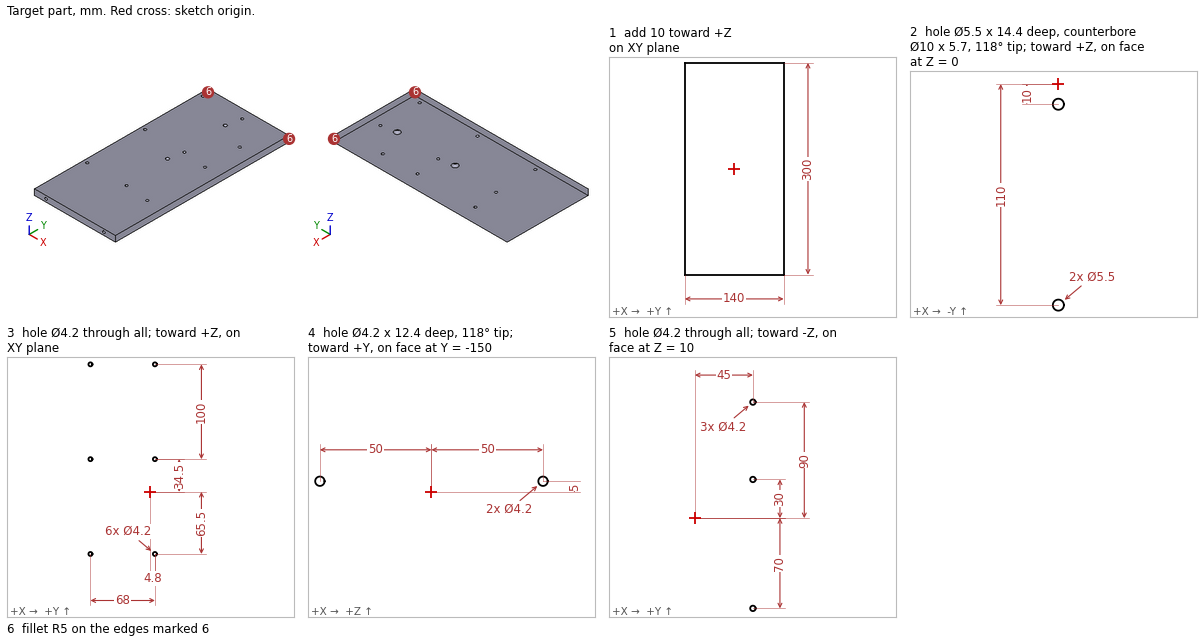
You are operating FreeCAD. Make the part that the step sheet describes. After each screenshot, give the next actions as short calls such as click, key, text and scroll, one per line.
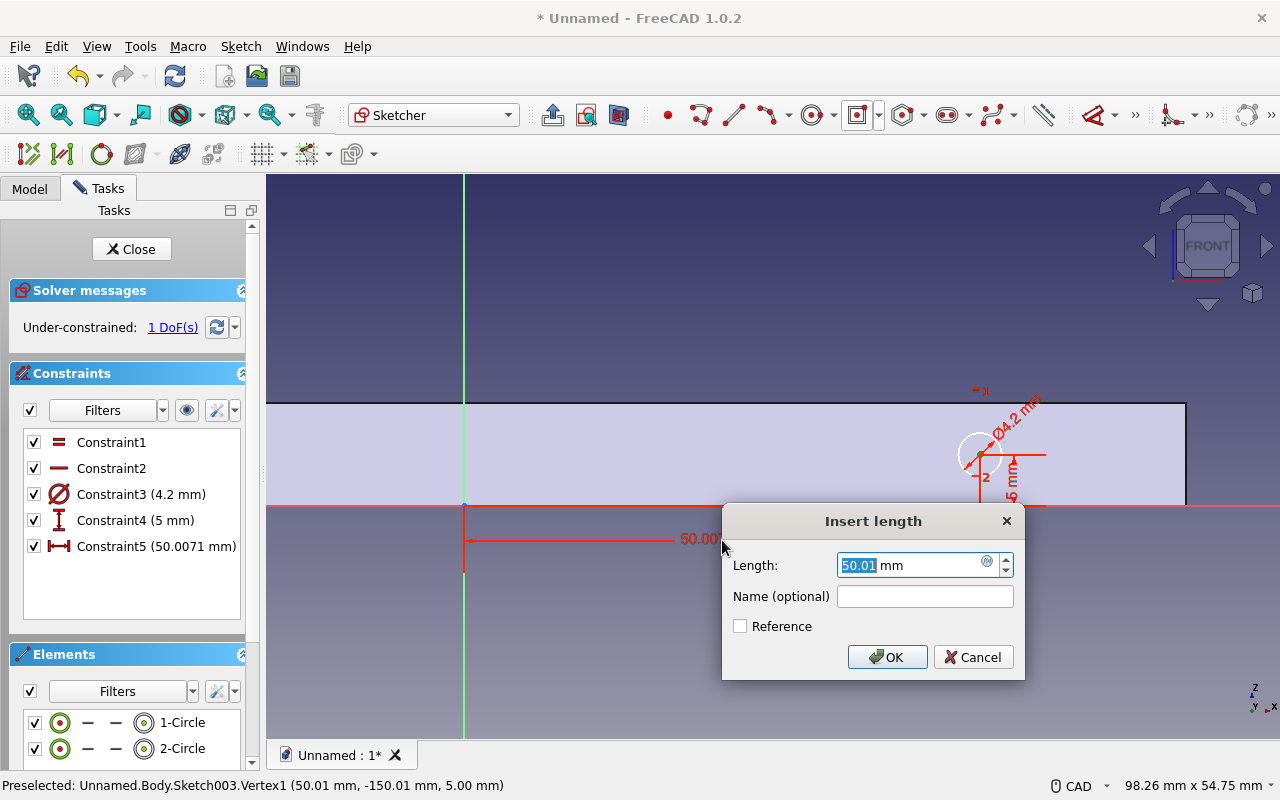
text(50)
key(Return)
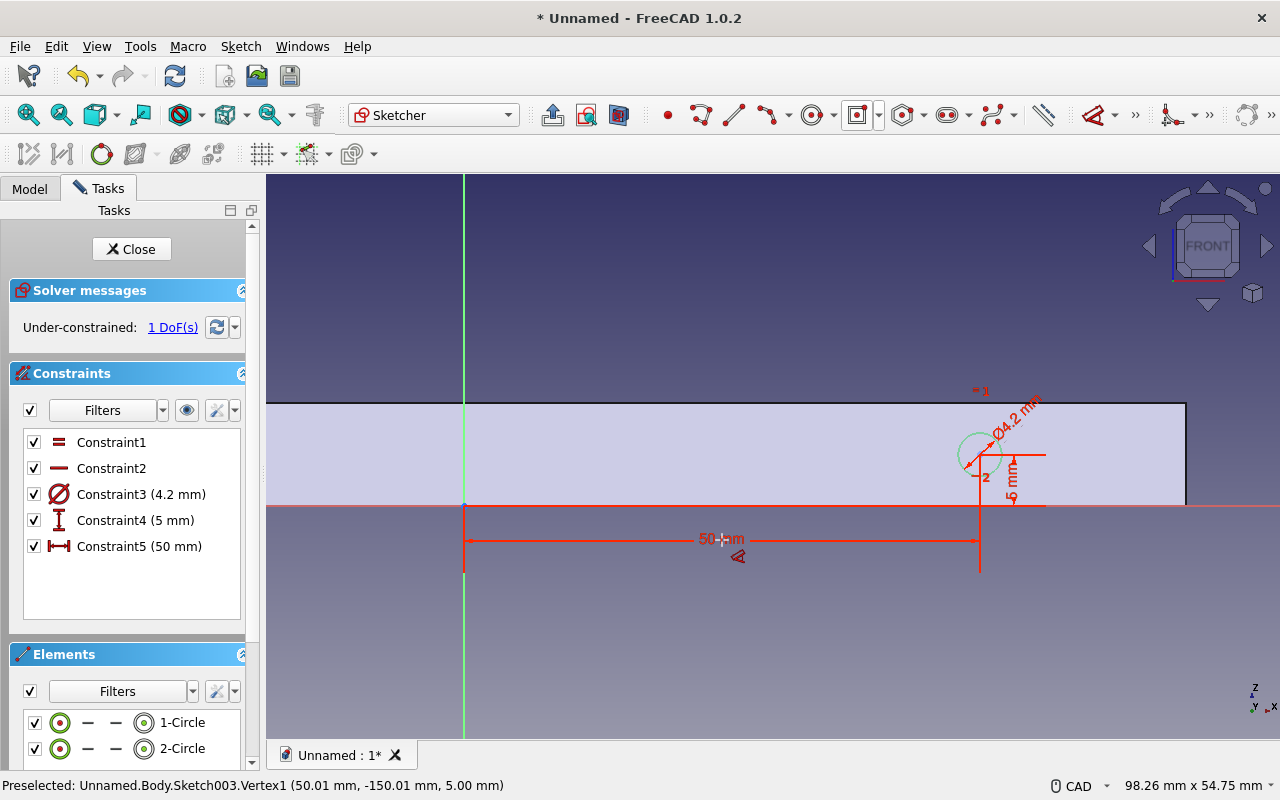
scroll(997, 440, down, 3)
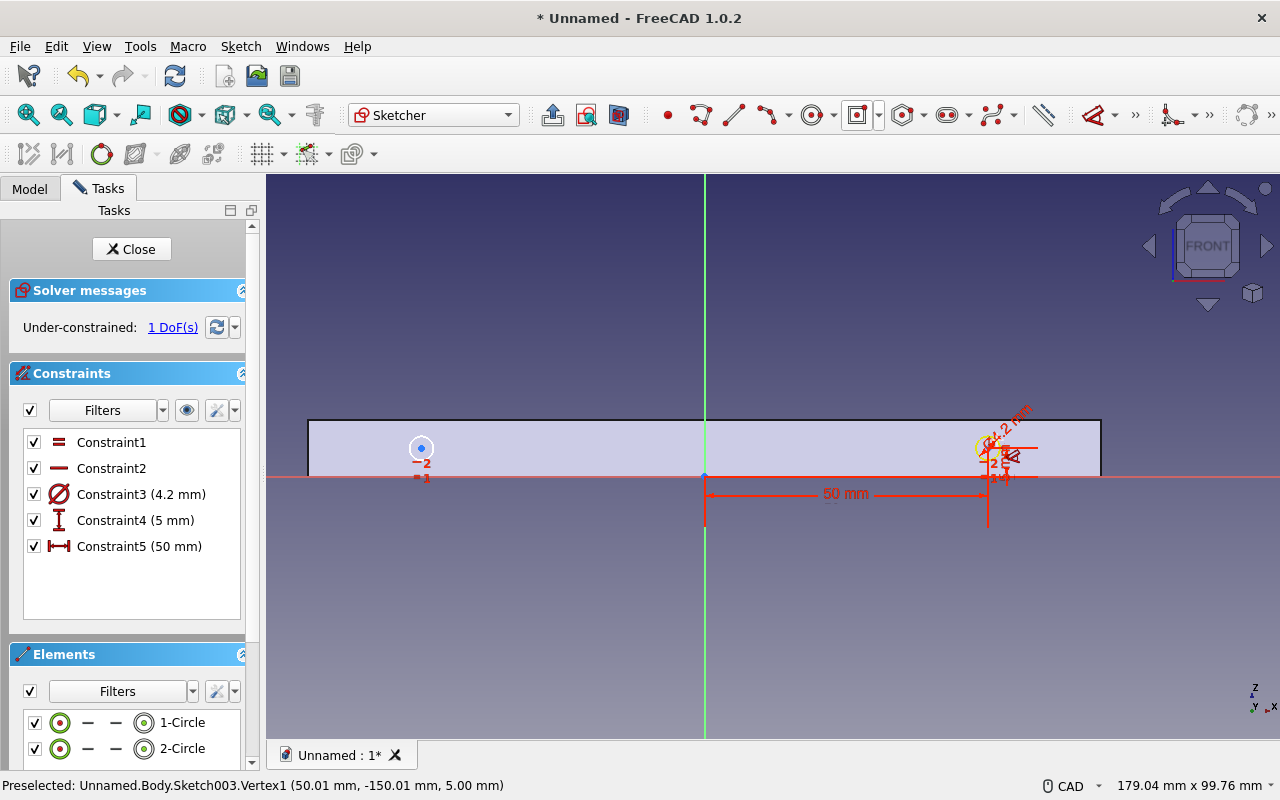
click(422, 448)
click(563, 511)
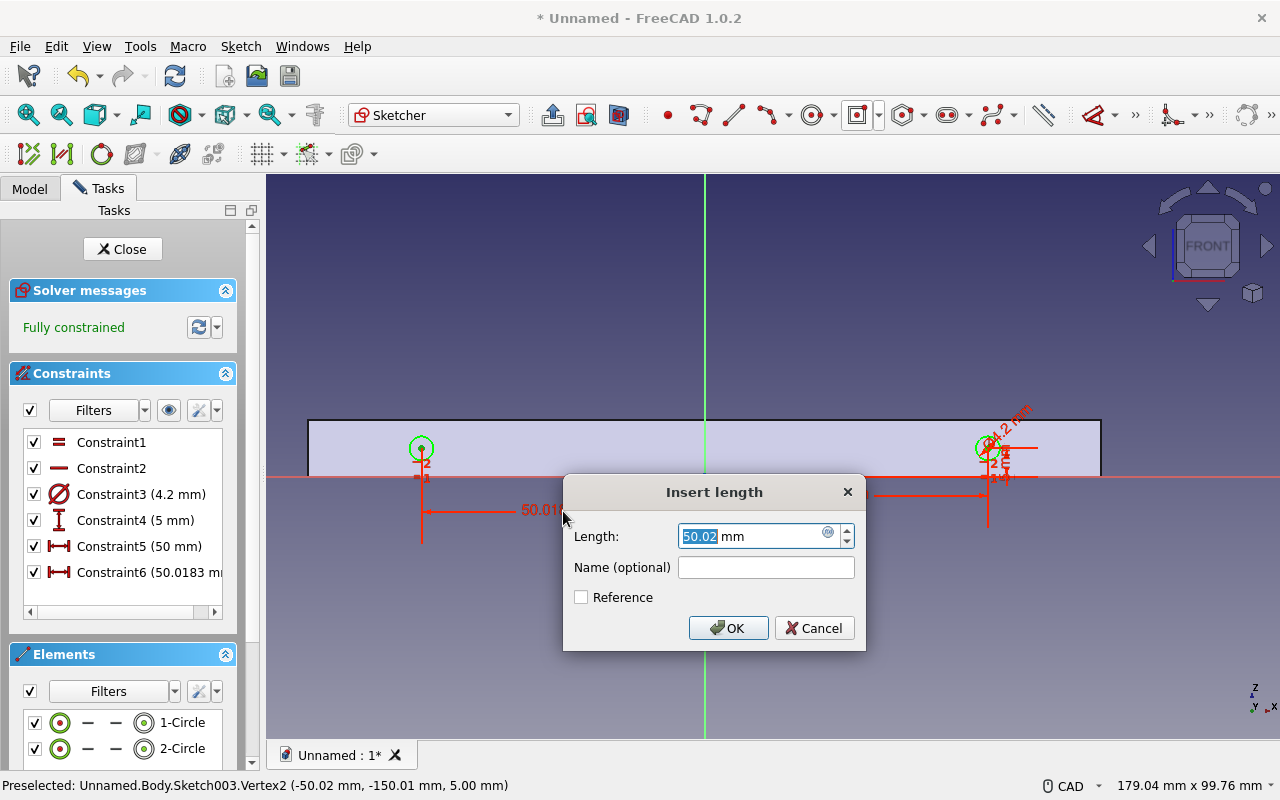
text(50)
key(Return)
key(Escape)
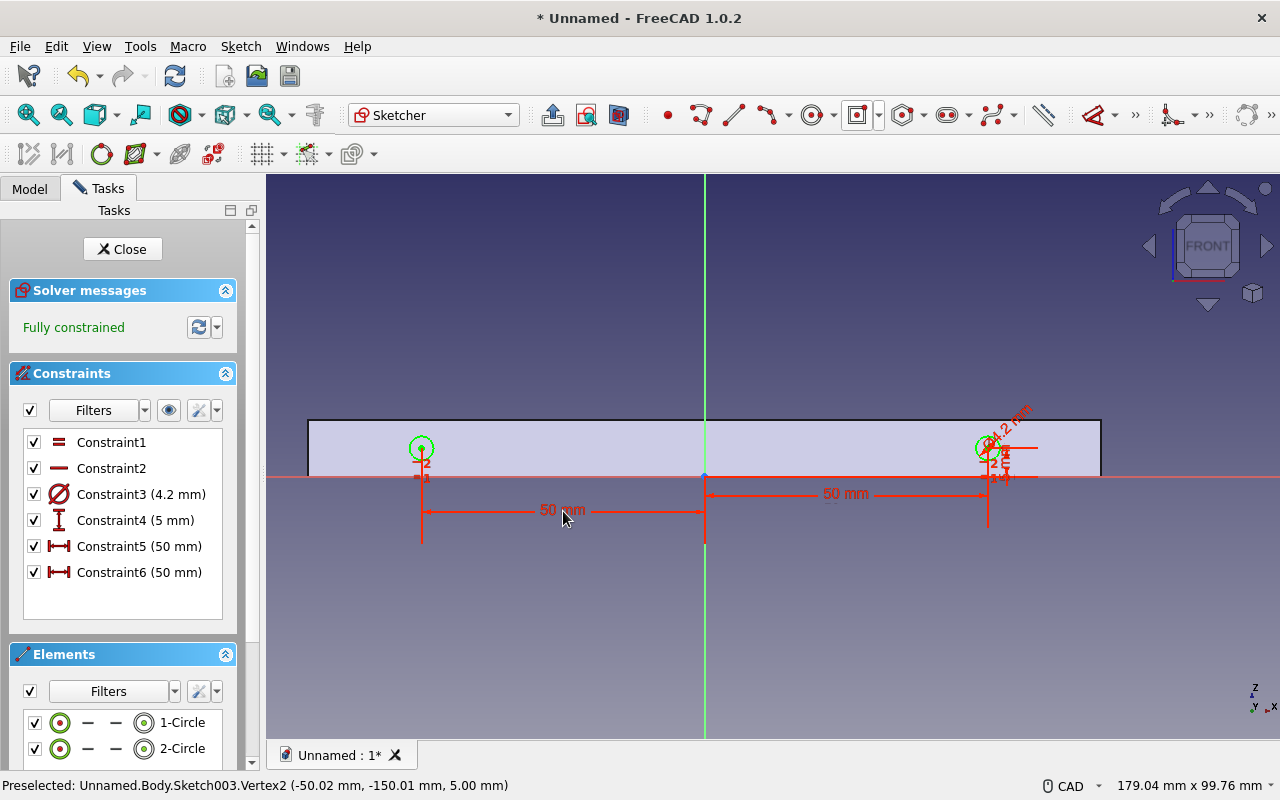
click(123, 249)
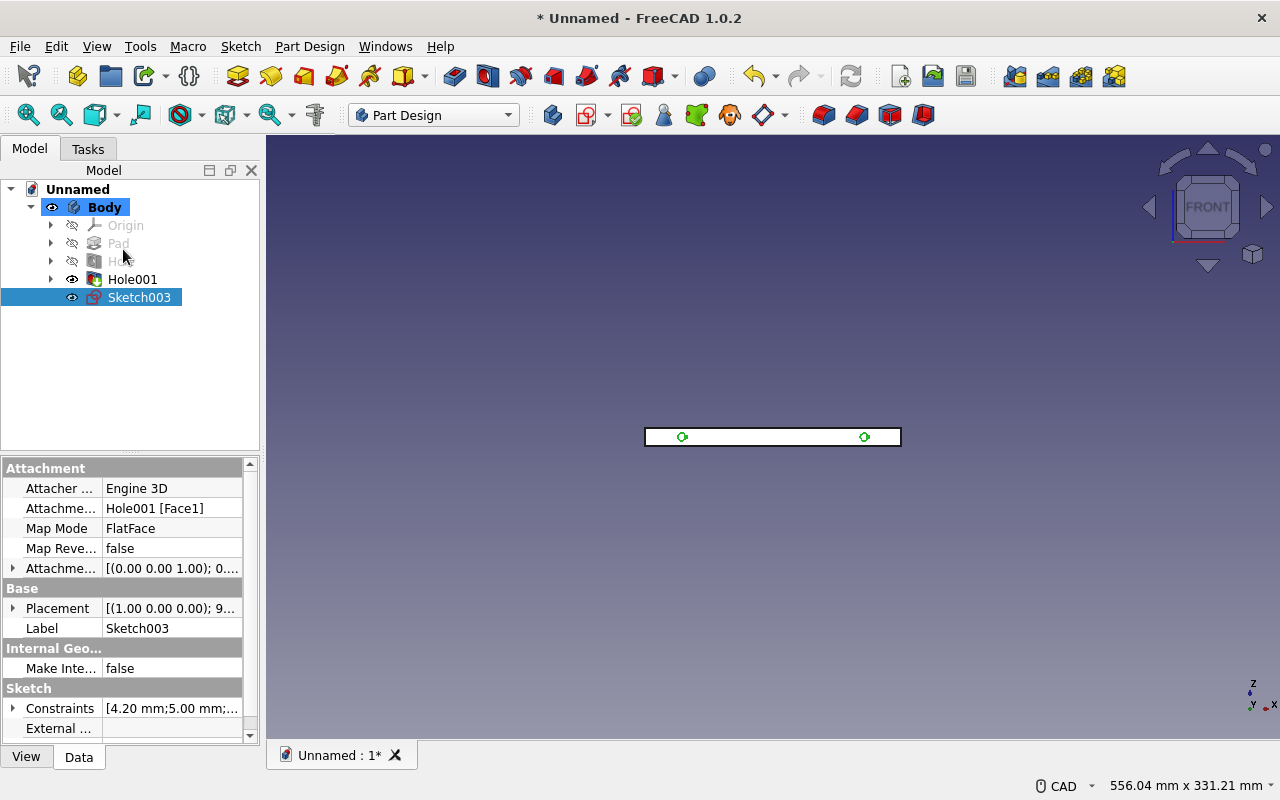
click(488, 76)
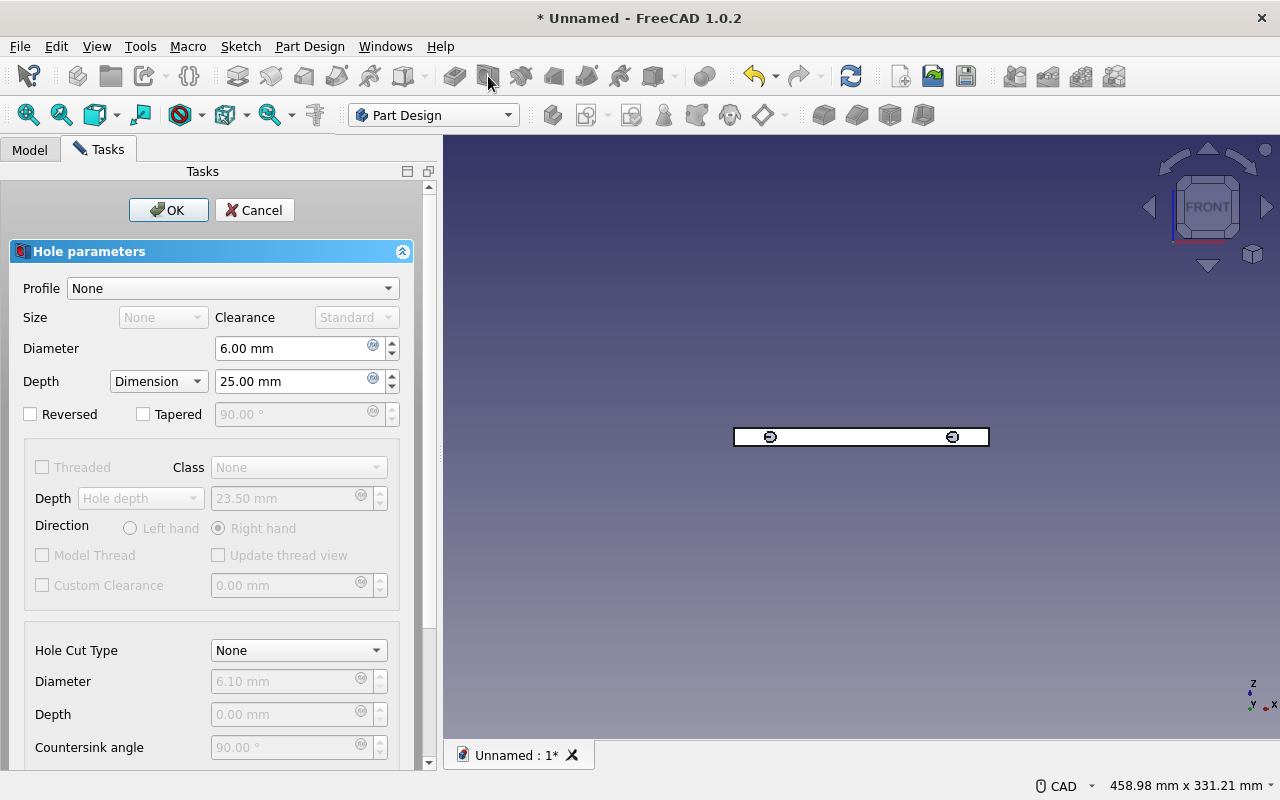
triple_click(300, 348)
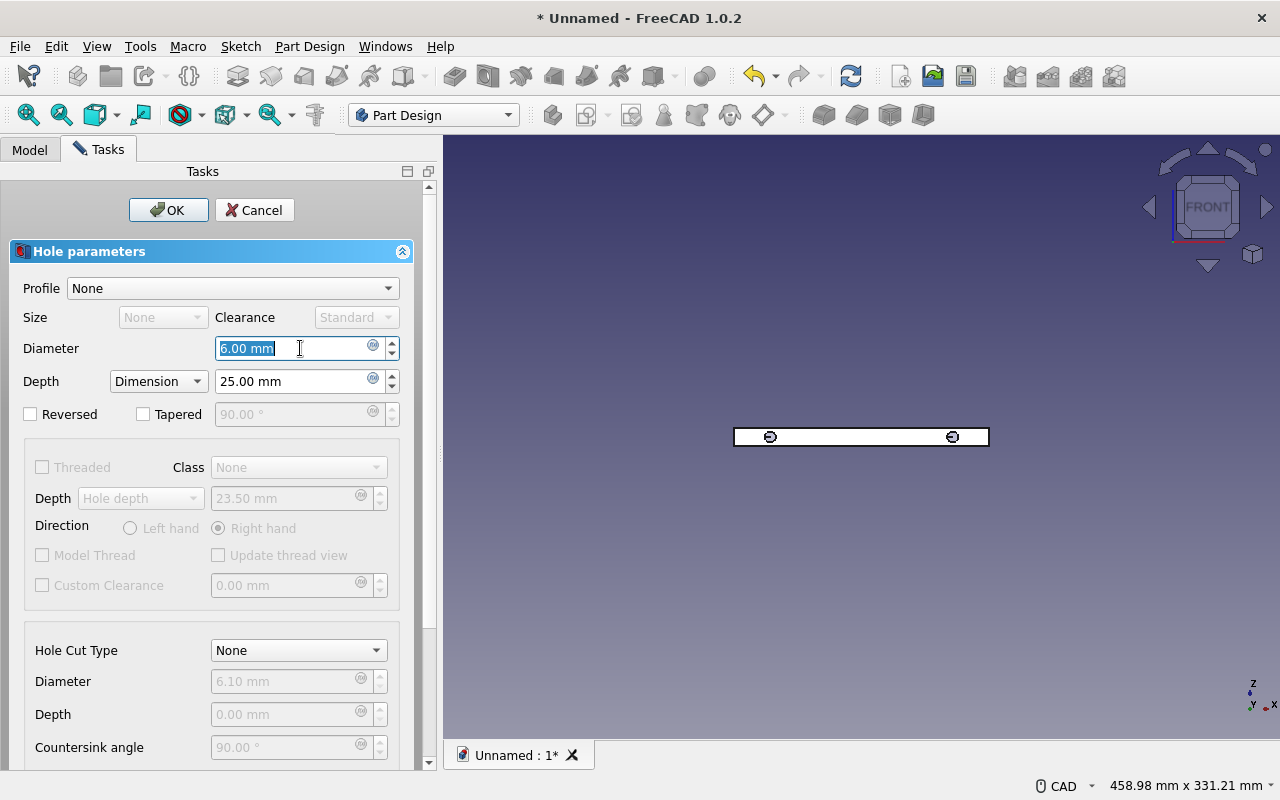
text(4.2)
key(Tab)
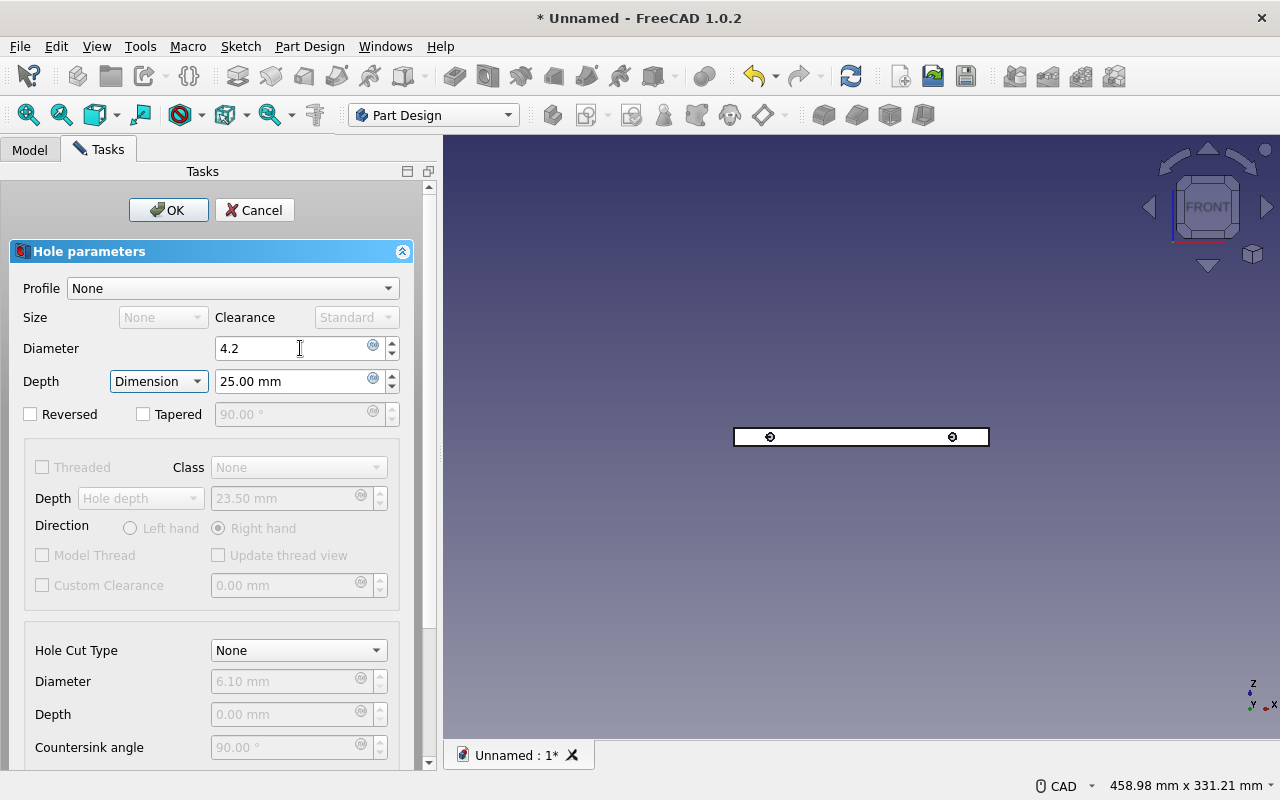
triple_click(300, 382)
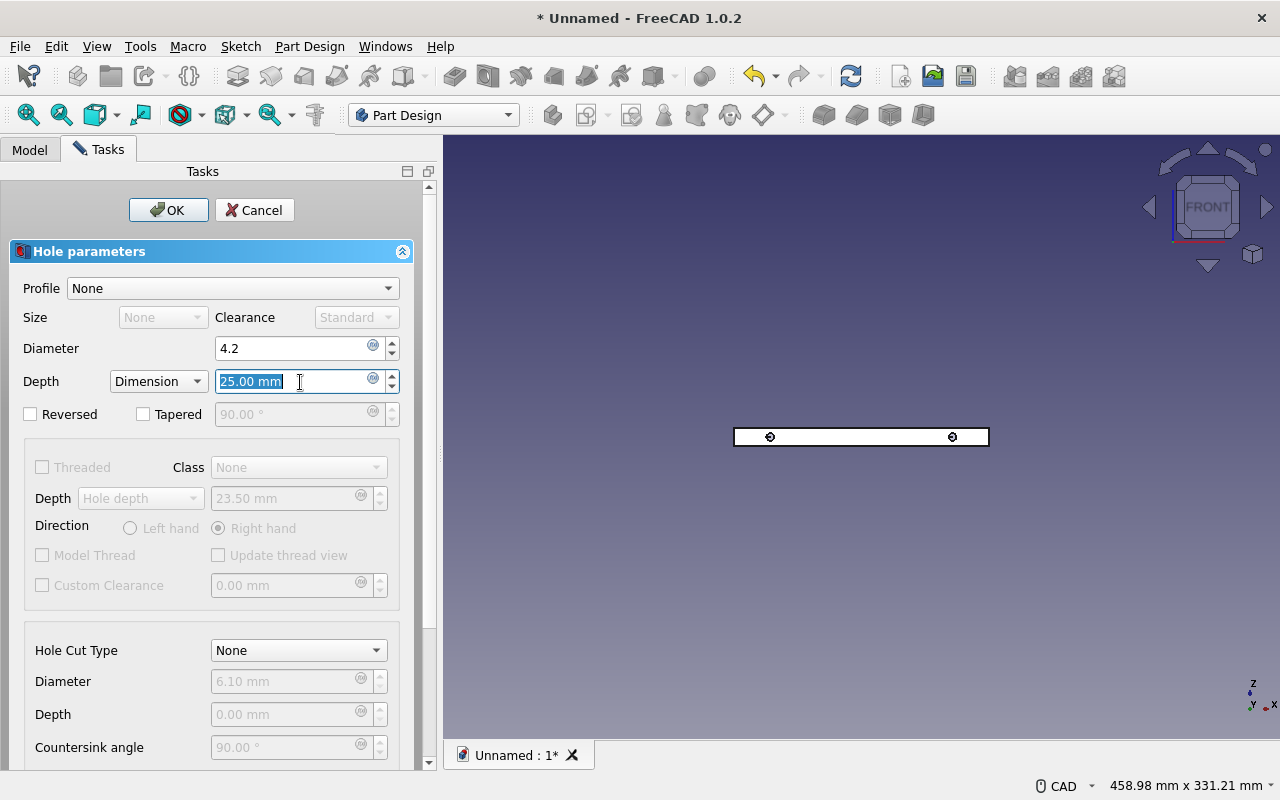
text(12.4)
key(Tab)